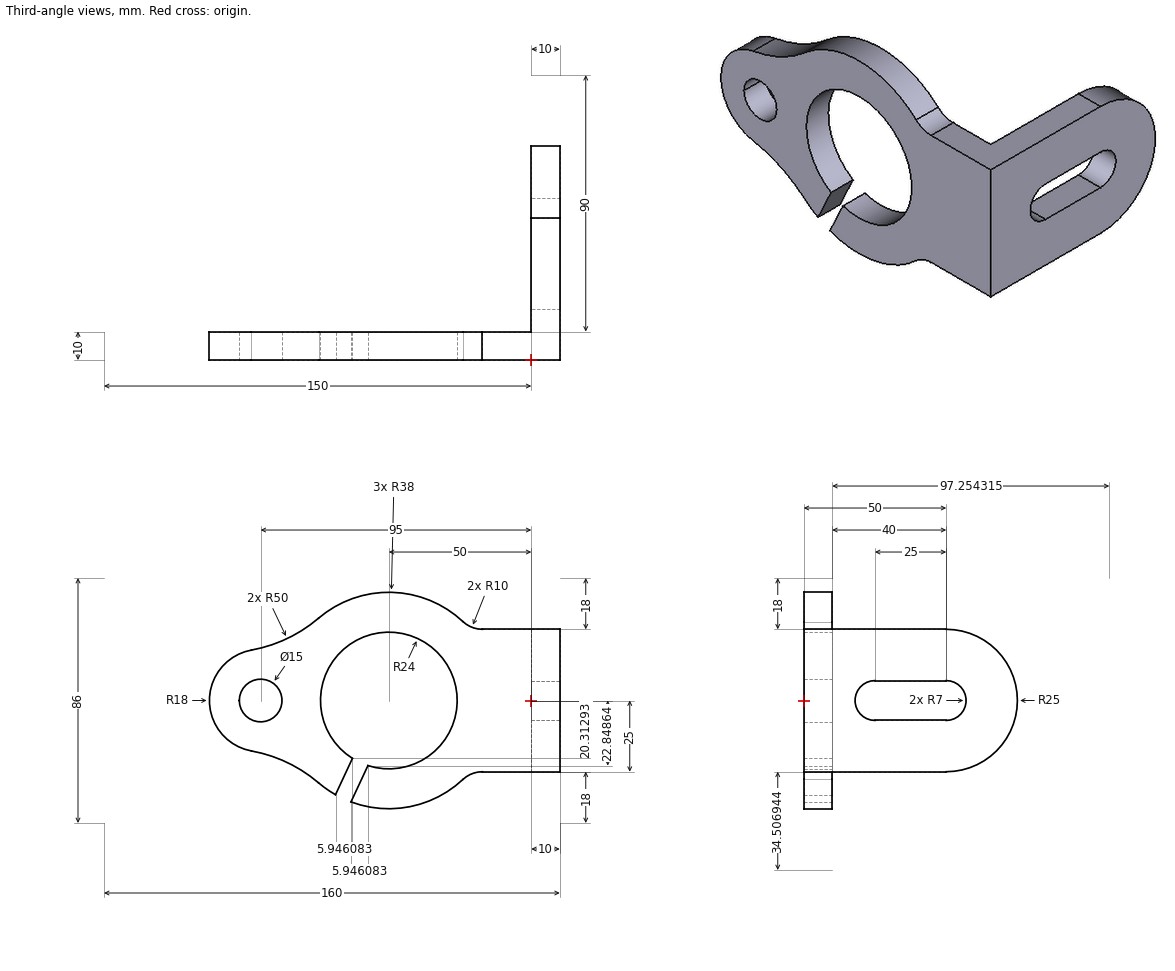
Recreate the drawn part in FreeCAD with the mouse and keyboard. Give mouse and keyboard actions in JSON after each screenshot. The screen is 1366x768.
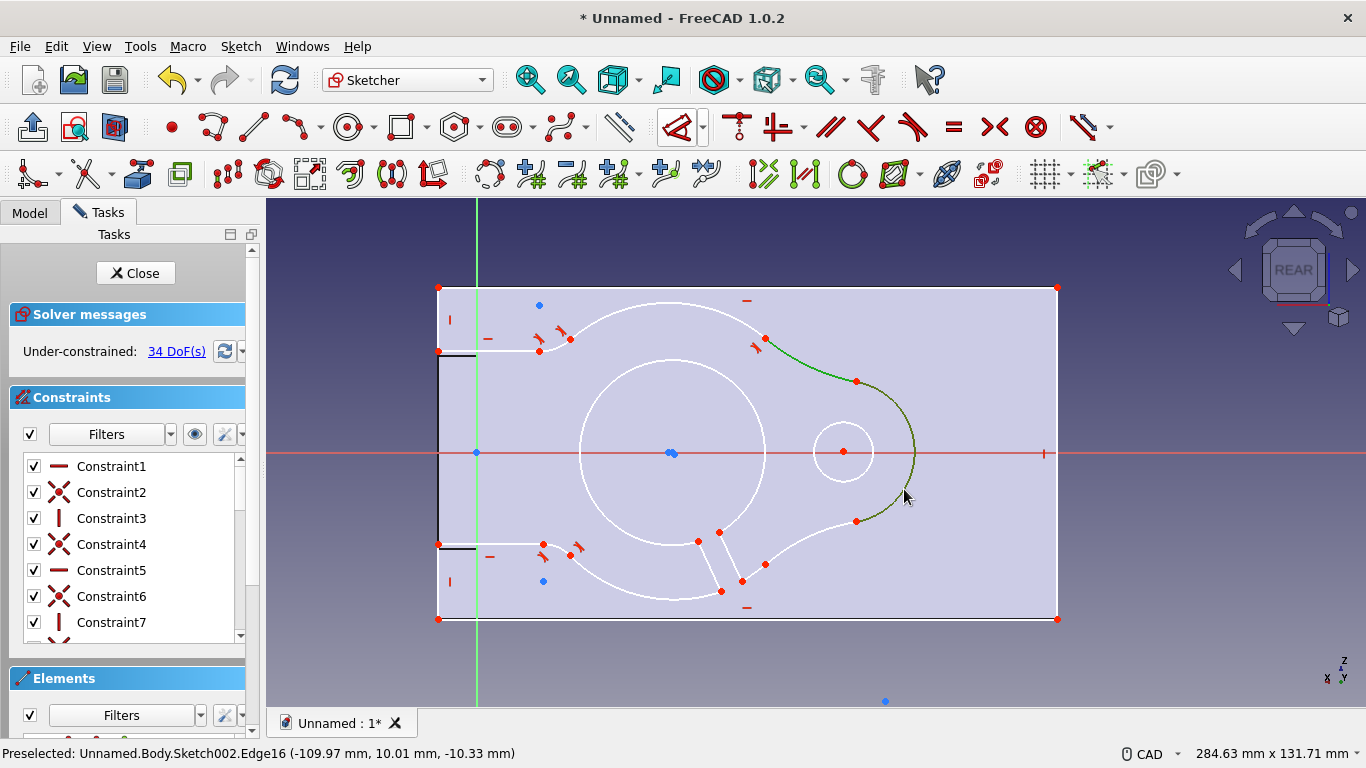
{"action": "key", "text": "t"}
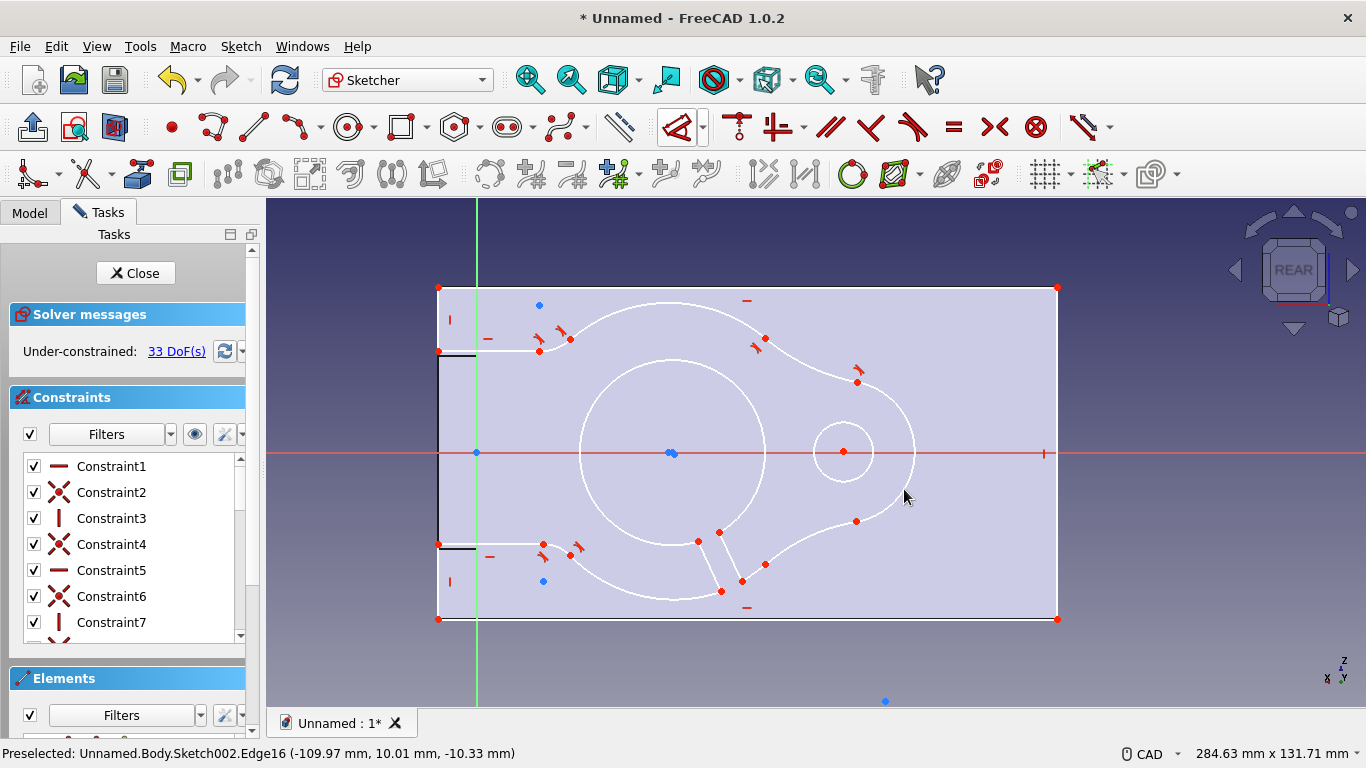
{"action": "left_click", "coordinate": [904, 490]}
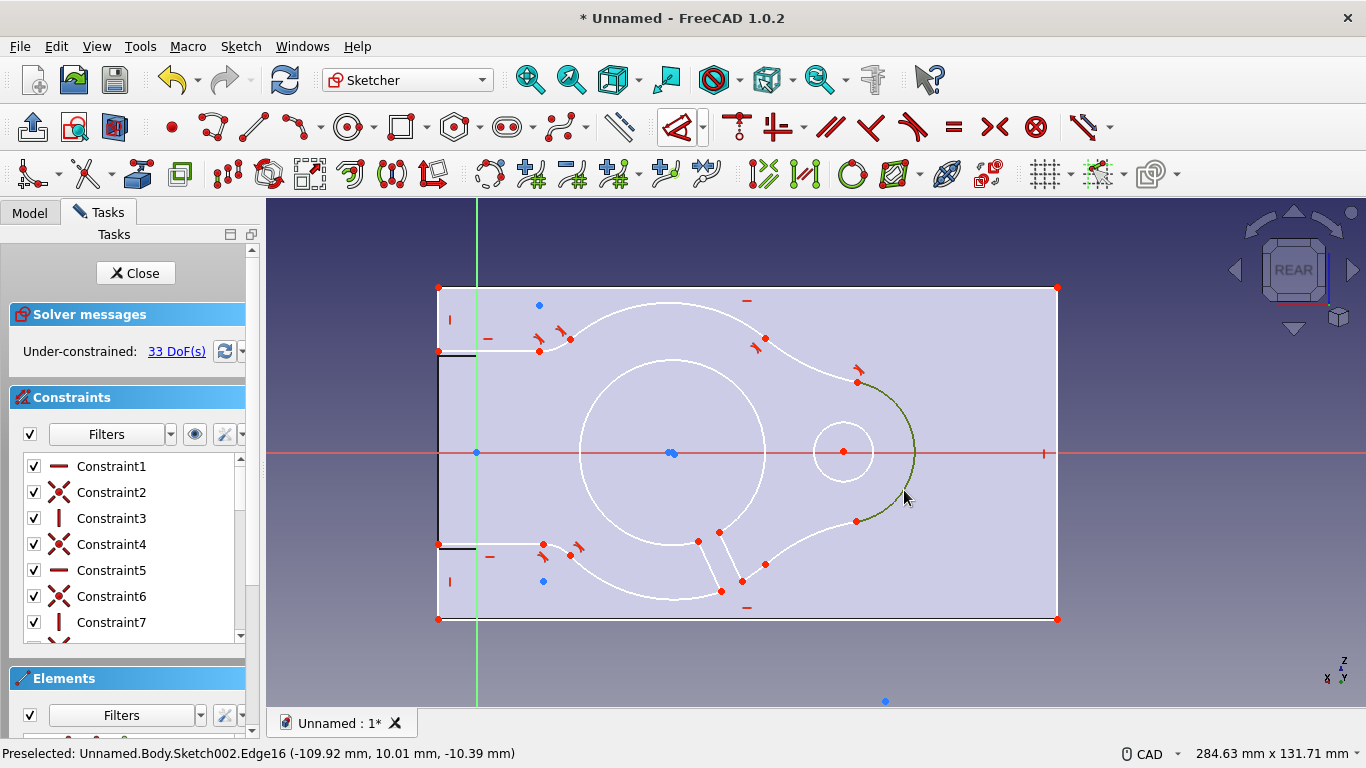
{"action": "left_click", "coordinate": [827, 529]}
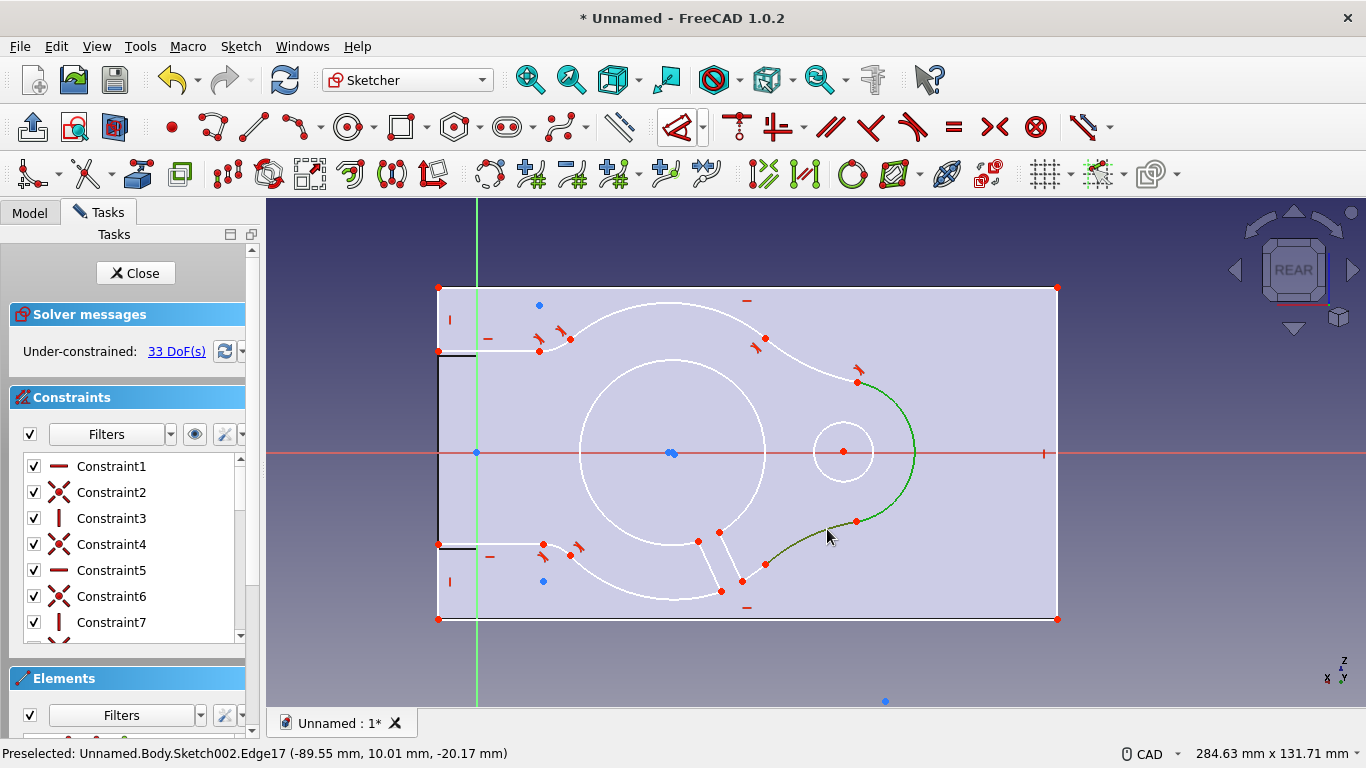
{"action": "left_click", "coordinate": [913, 128]}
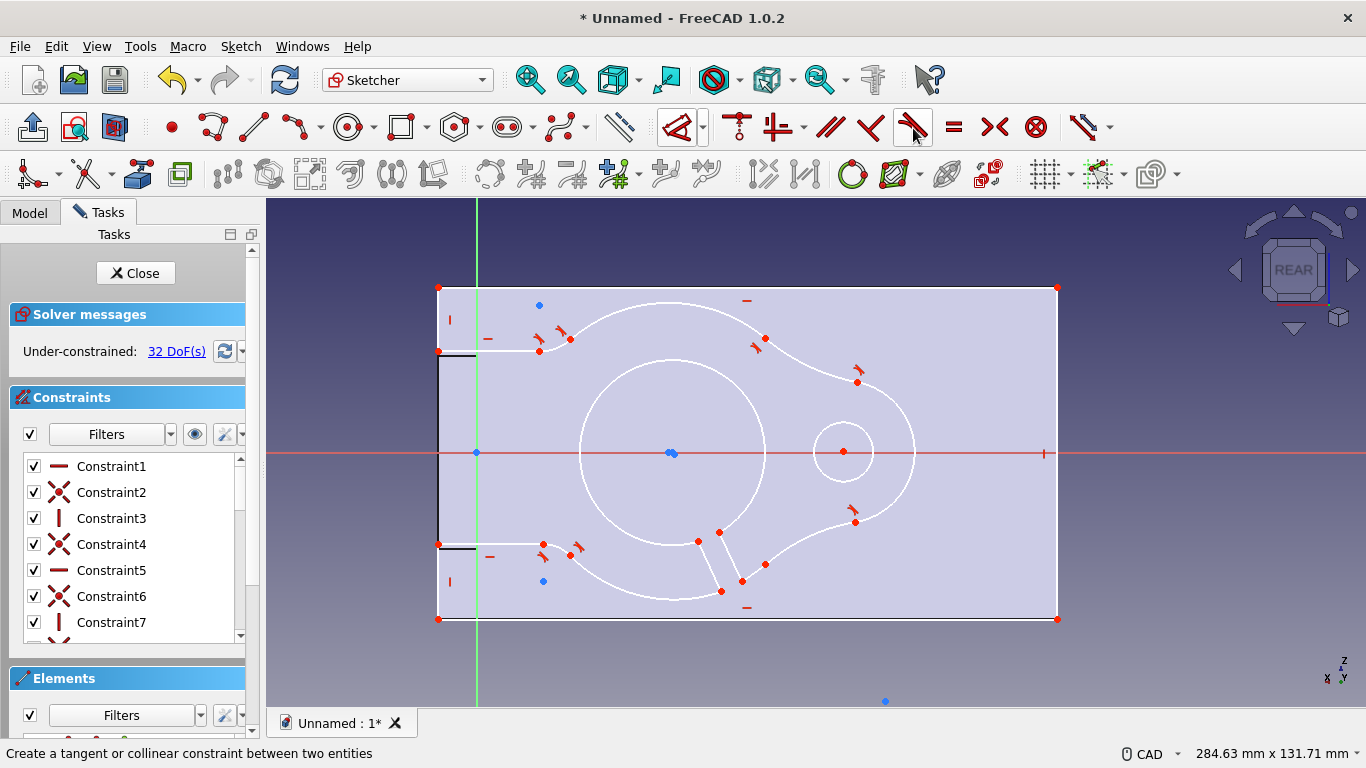
{"action": "left_click", "coordinate": [826, 530]}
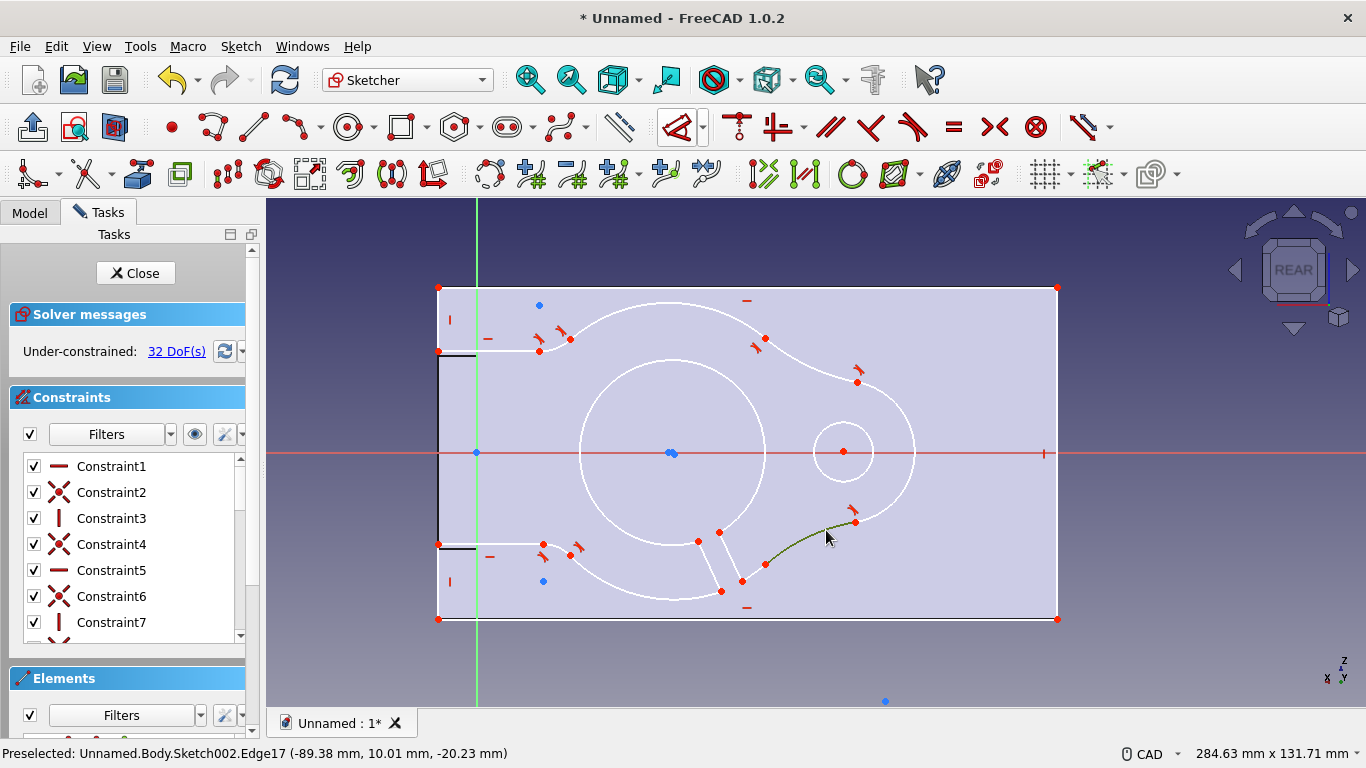
{"action": "left_click", "coordinate": [754, 573]}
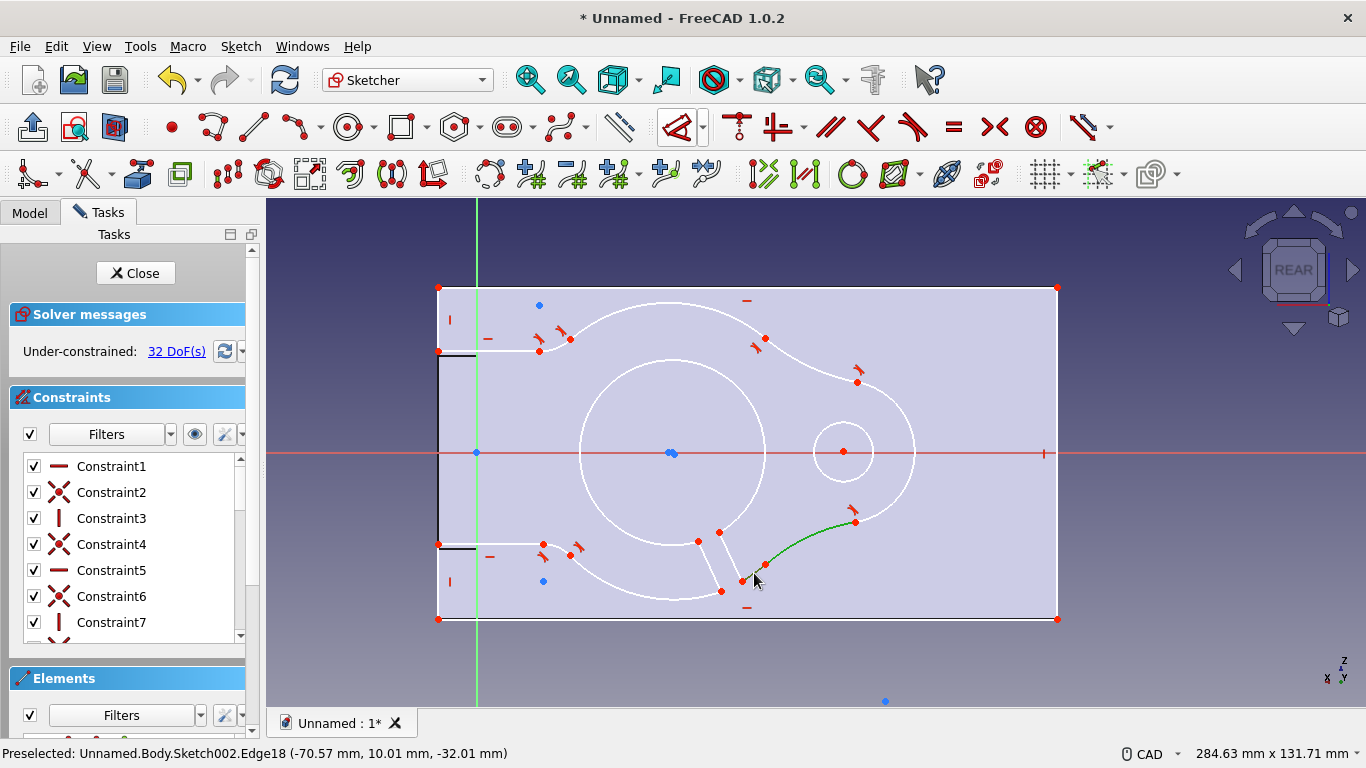
{"action": "left_click", "coordinate": [913, 128]}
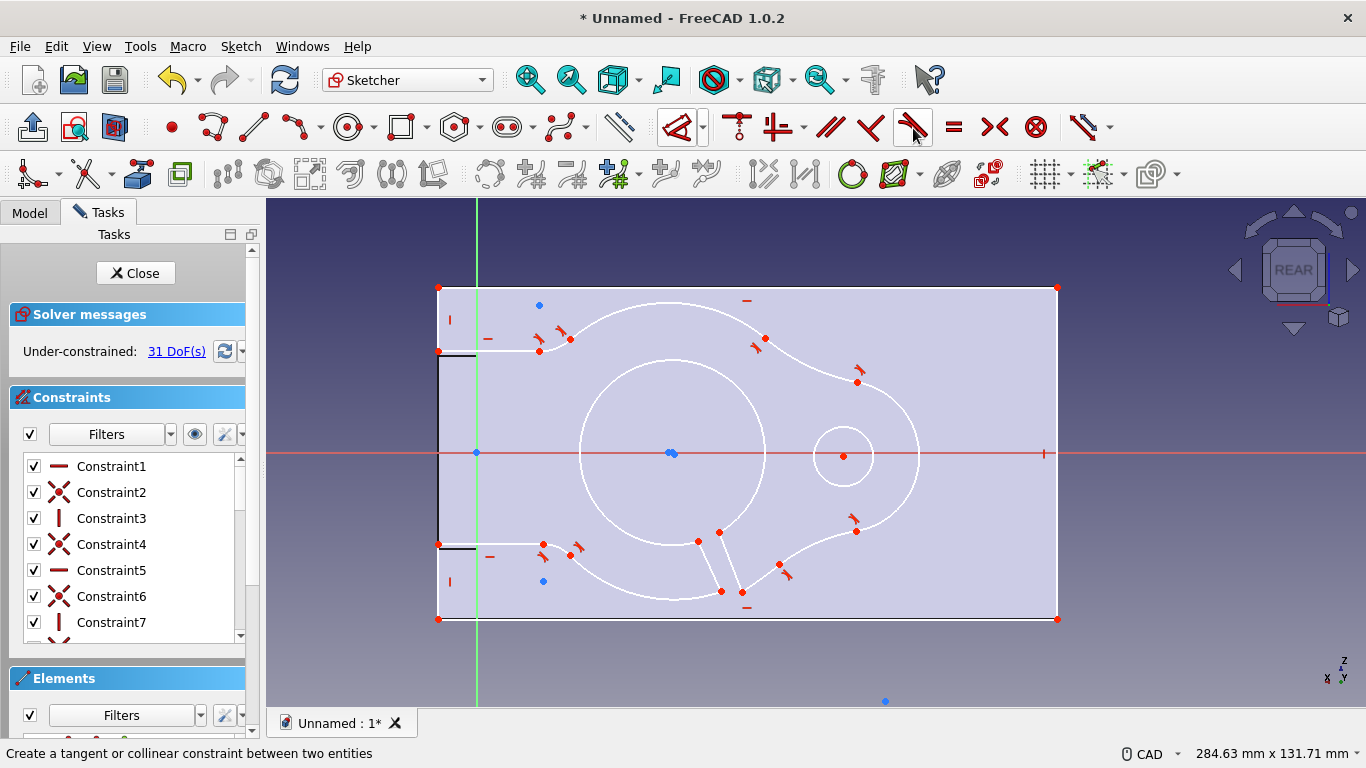
{"action": "left_click", "coordinate": [739, 388]}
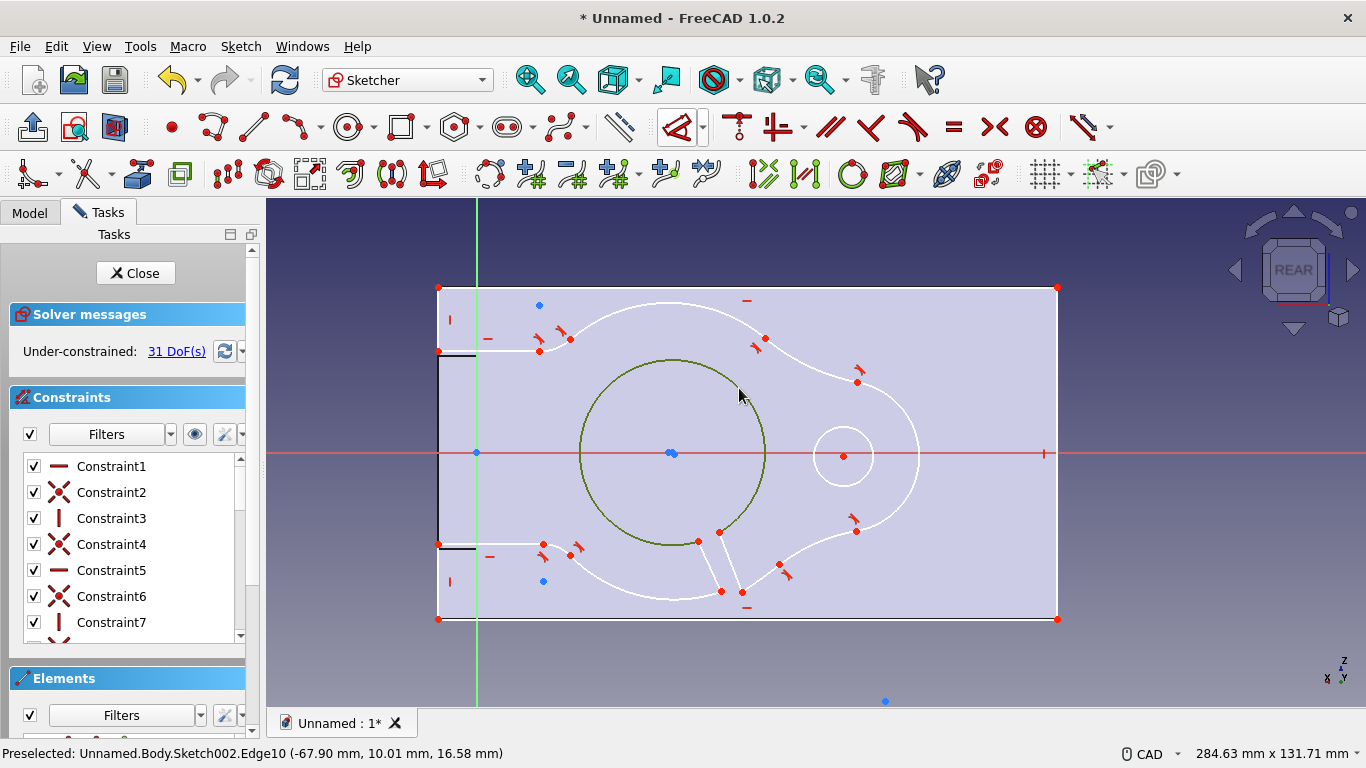
{"action": "left_click", "coordinate": [610, 584]}